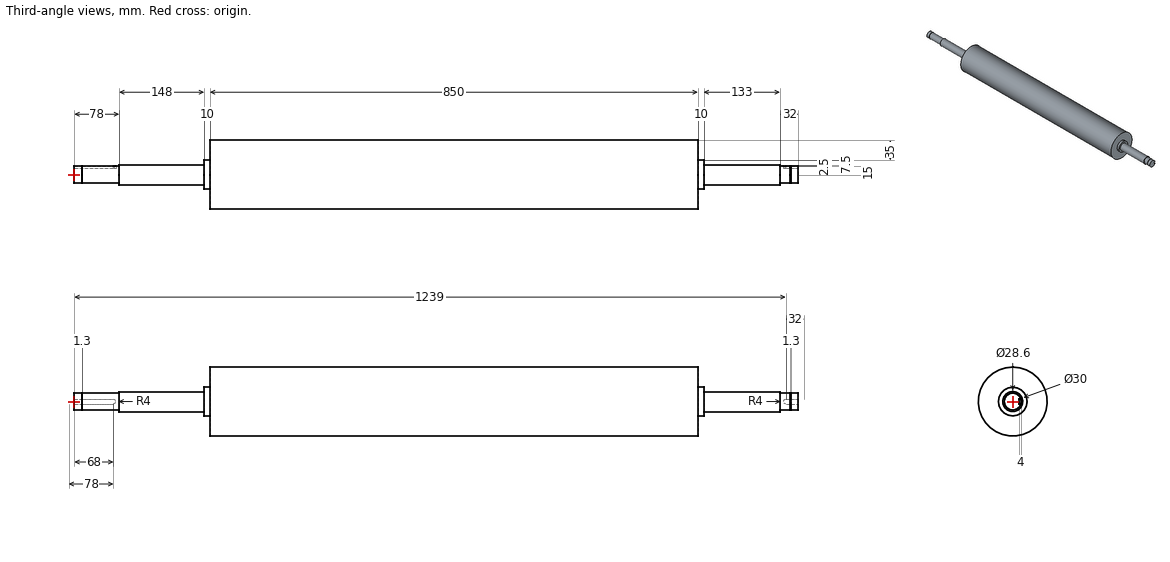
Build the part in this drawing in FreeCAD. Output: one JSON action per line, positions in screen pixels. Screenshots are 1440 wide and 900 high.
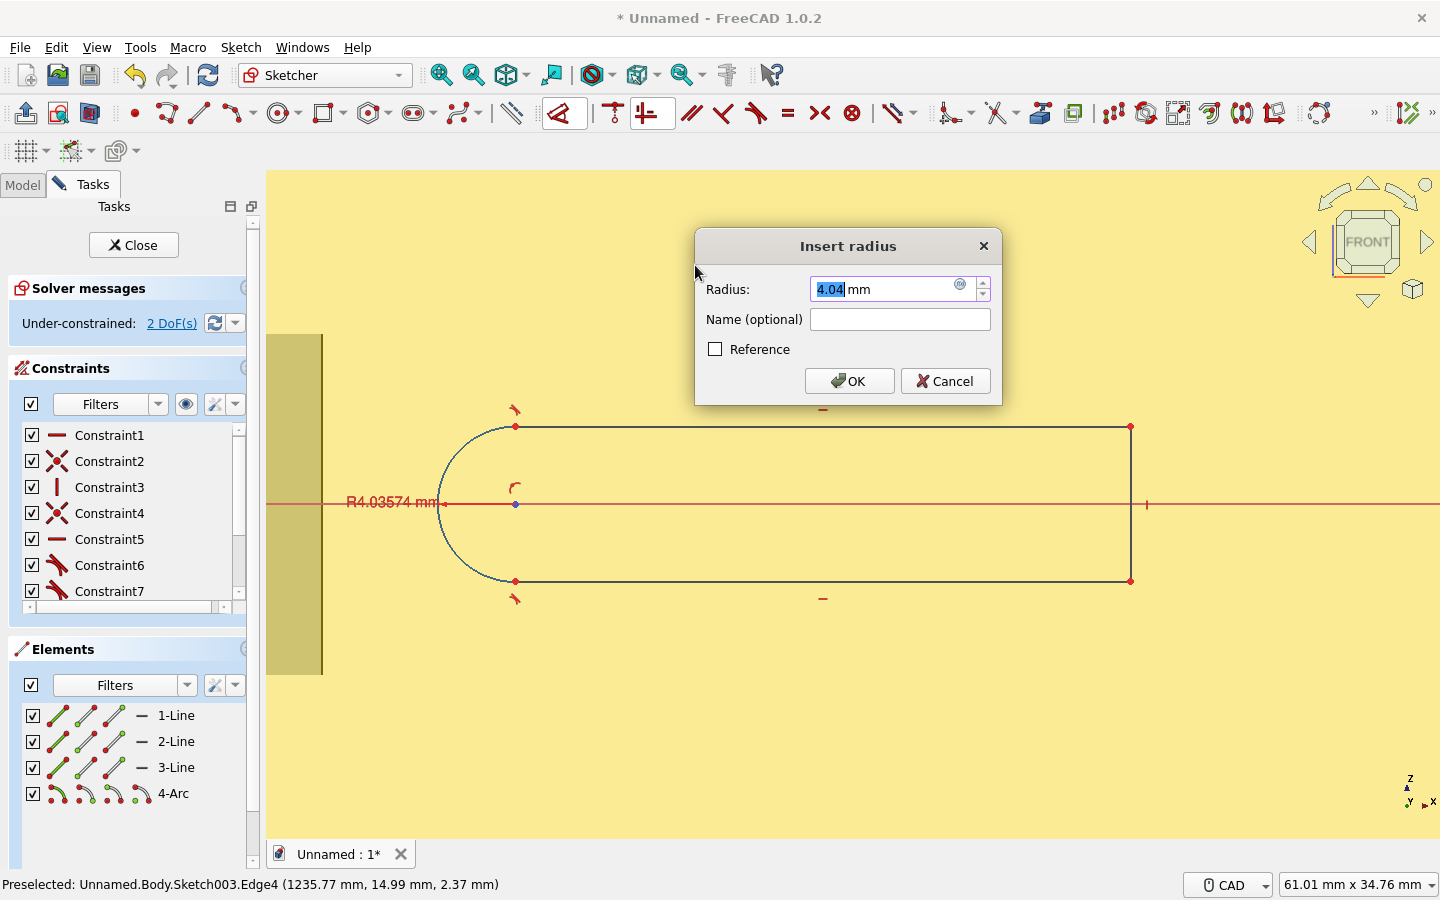
{"action": "type", "text": "4"}
{"action": "key", "text": "Return"}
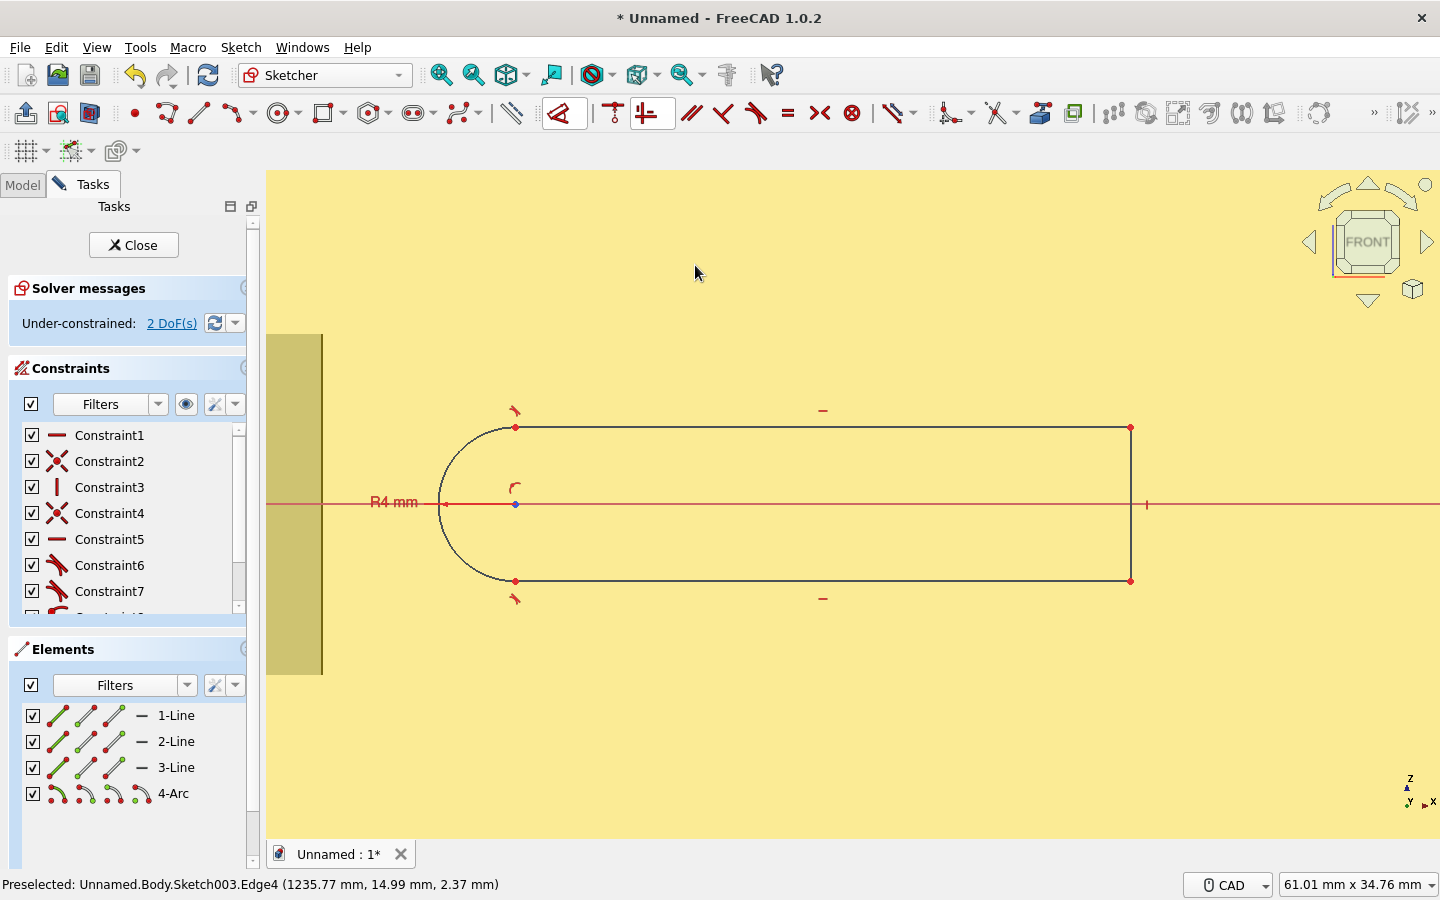
{"action": "left_click", "coordinate": [700, 427]}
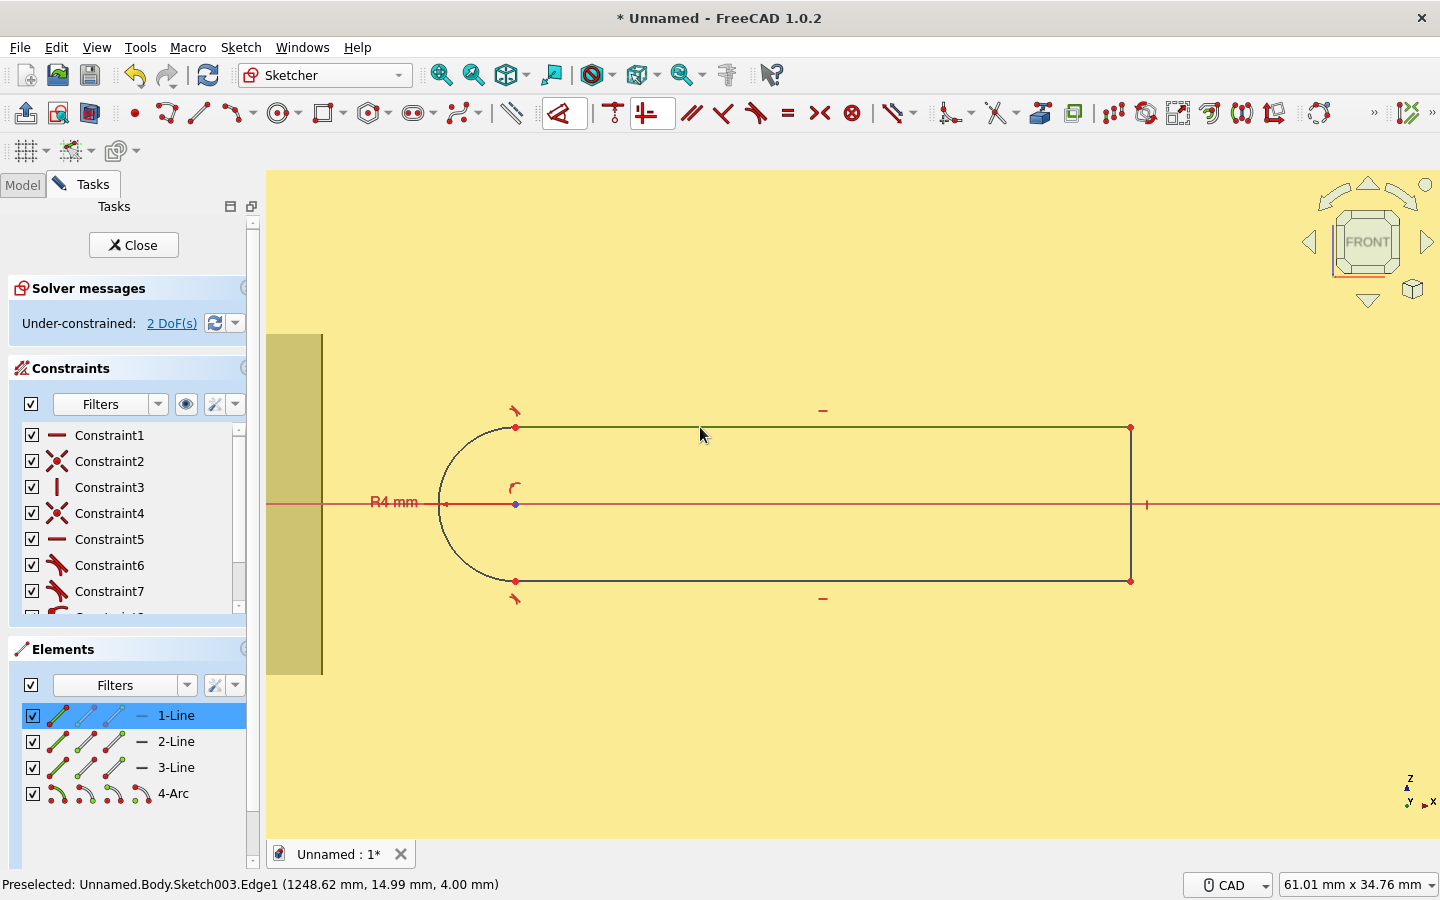
{"action": "key", "text": "l"}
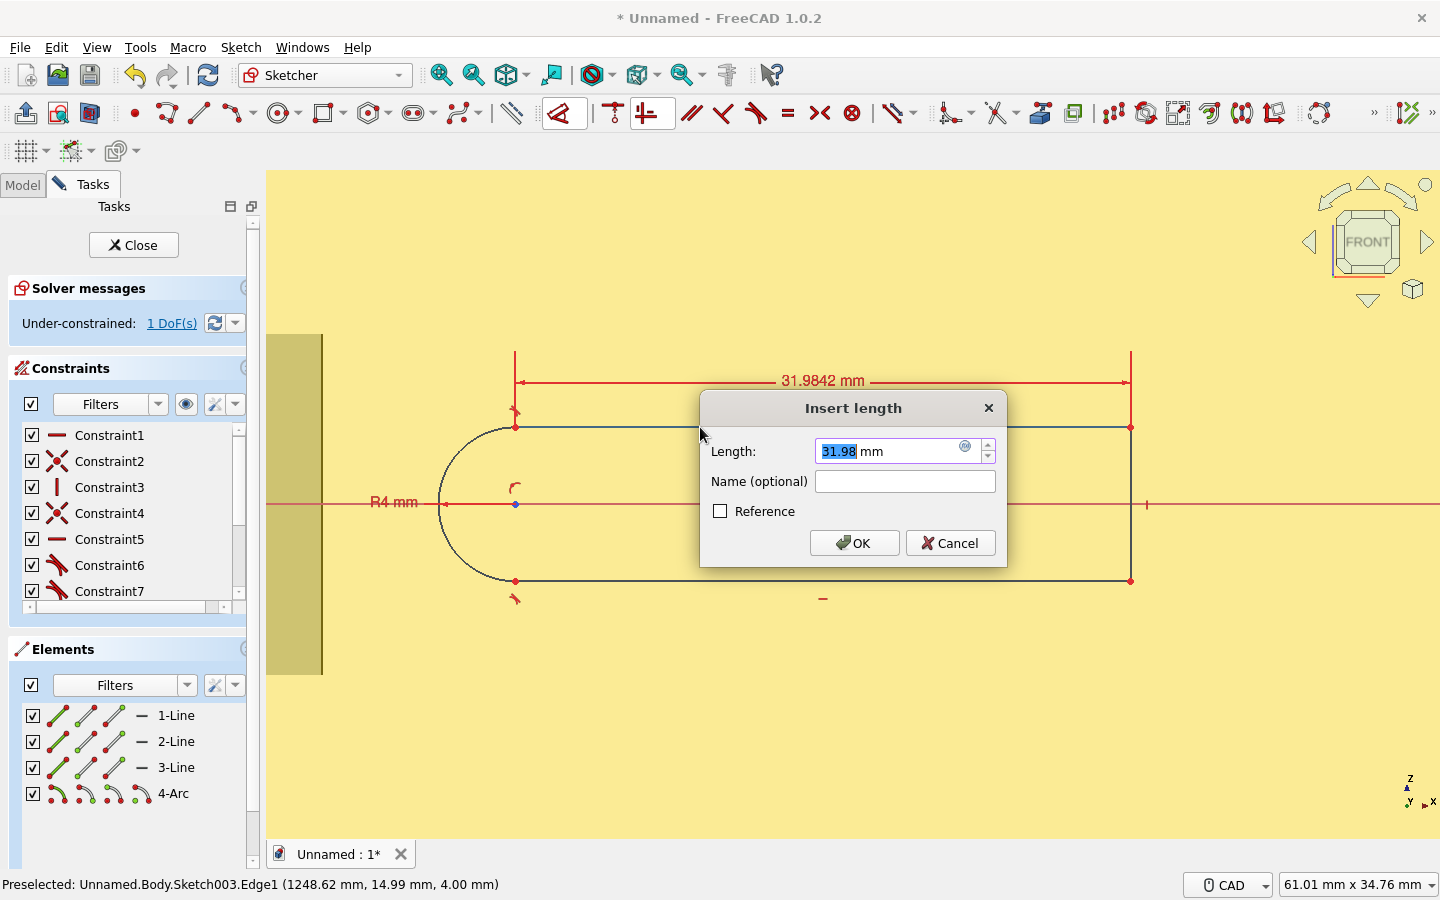
{"action": "type", "text": "32"}
{"action": "key", "text": "Return"}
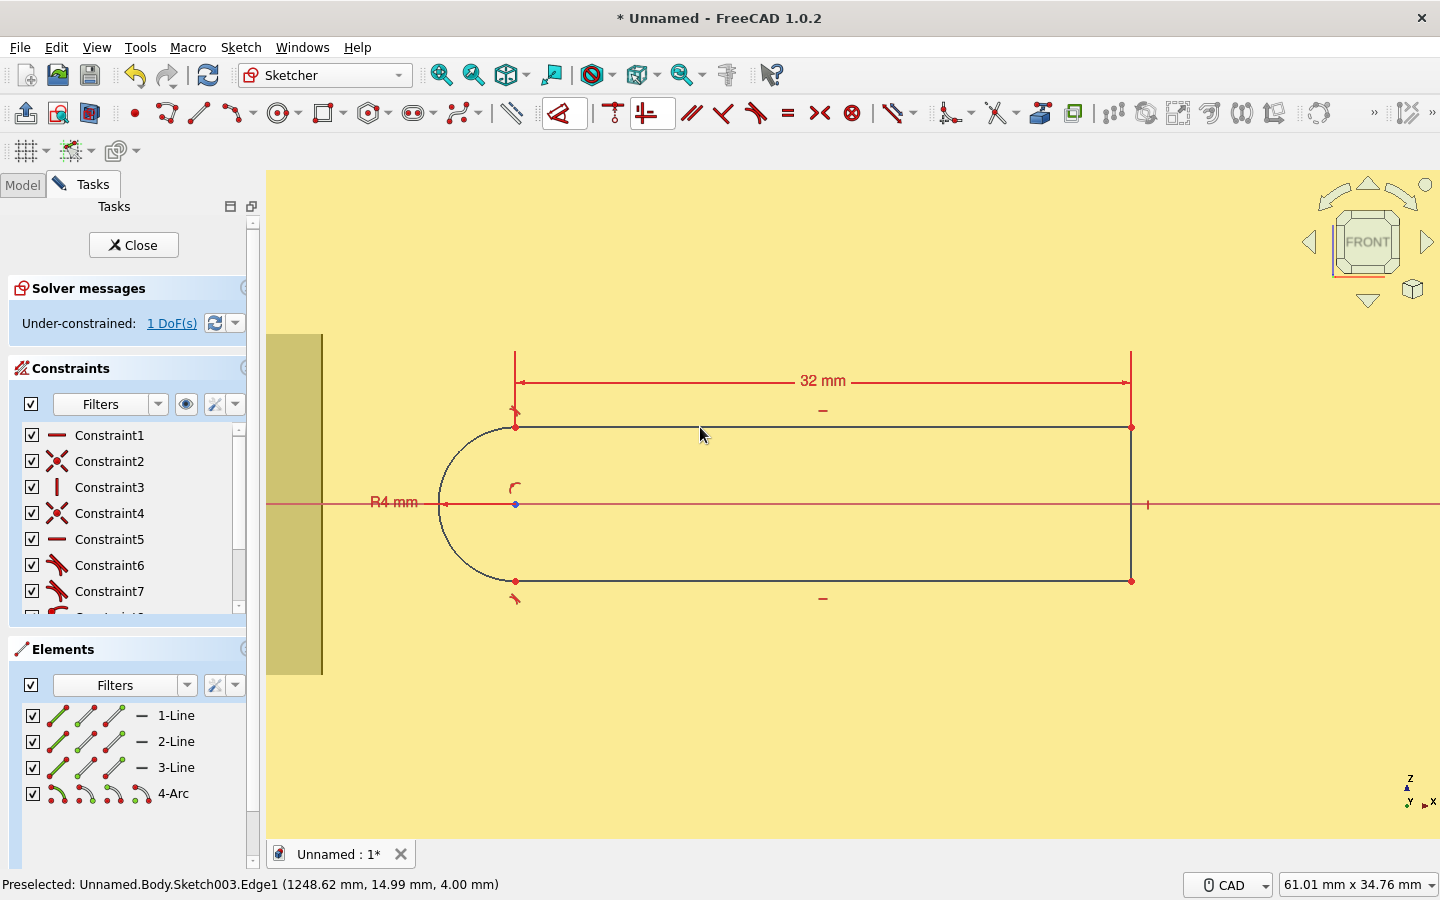
{"action": "left_click", "coordinate": [515, 427]}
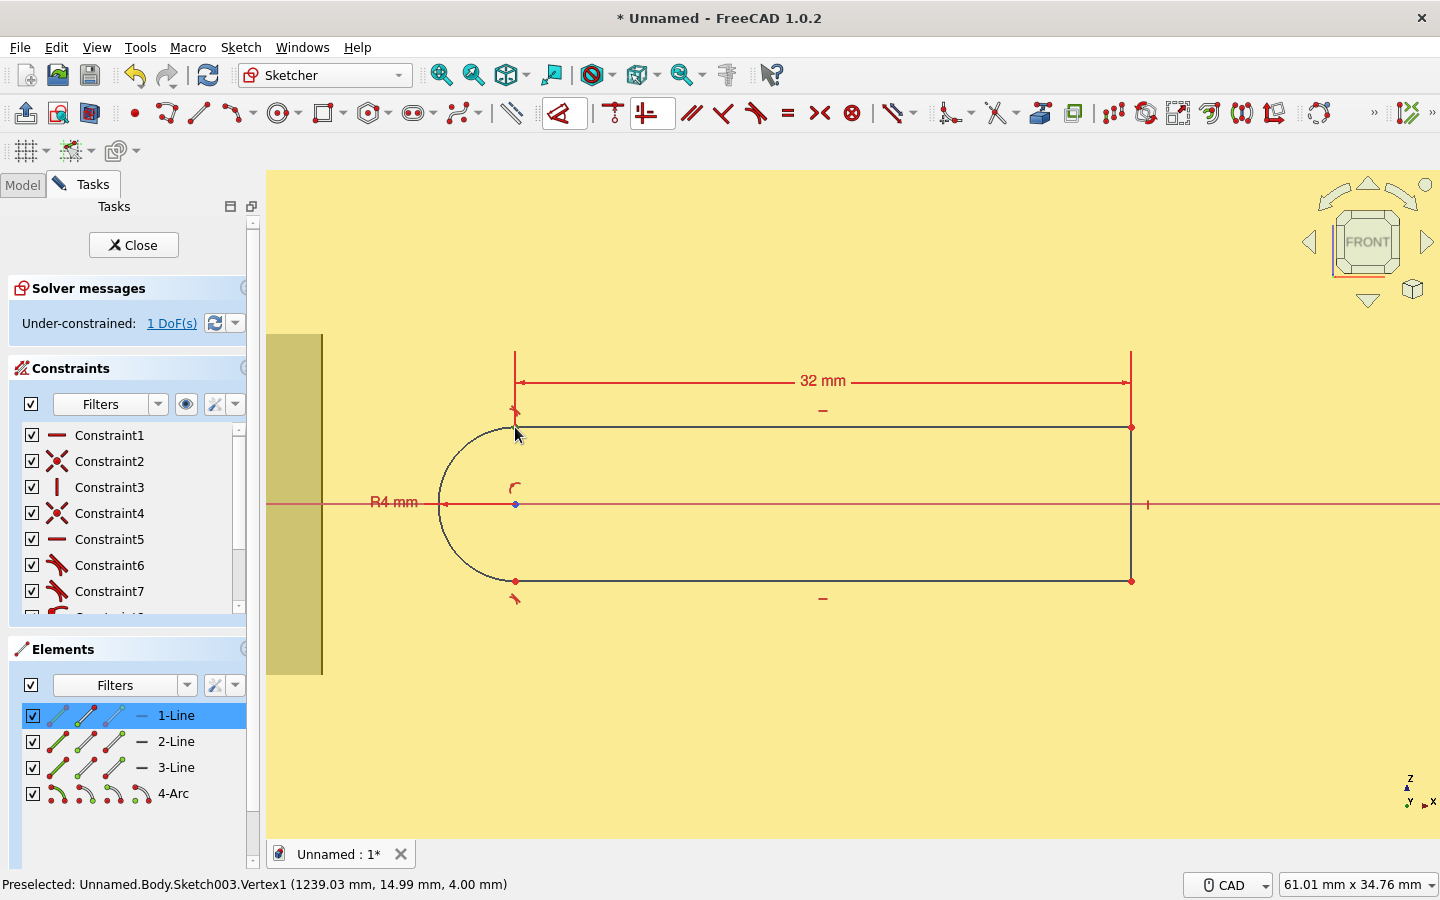
{"action": "key", "text": "l"}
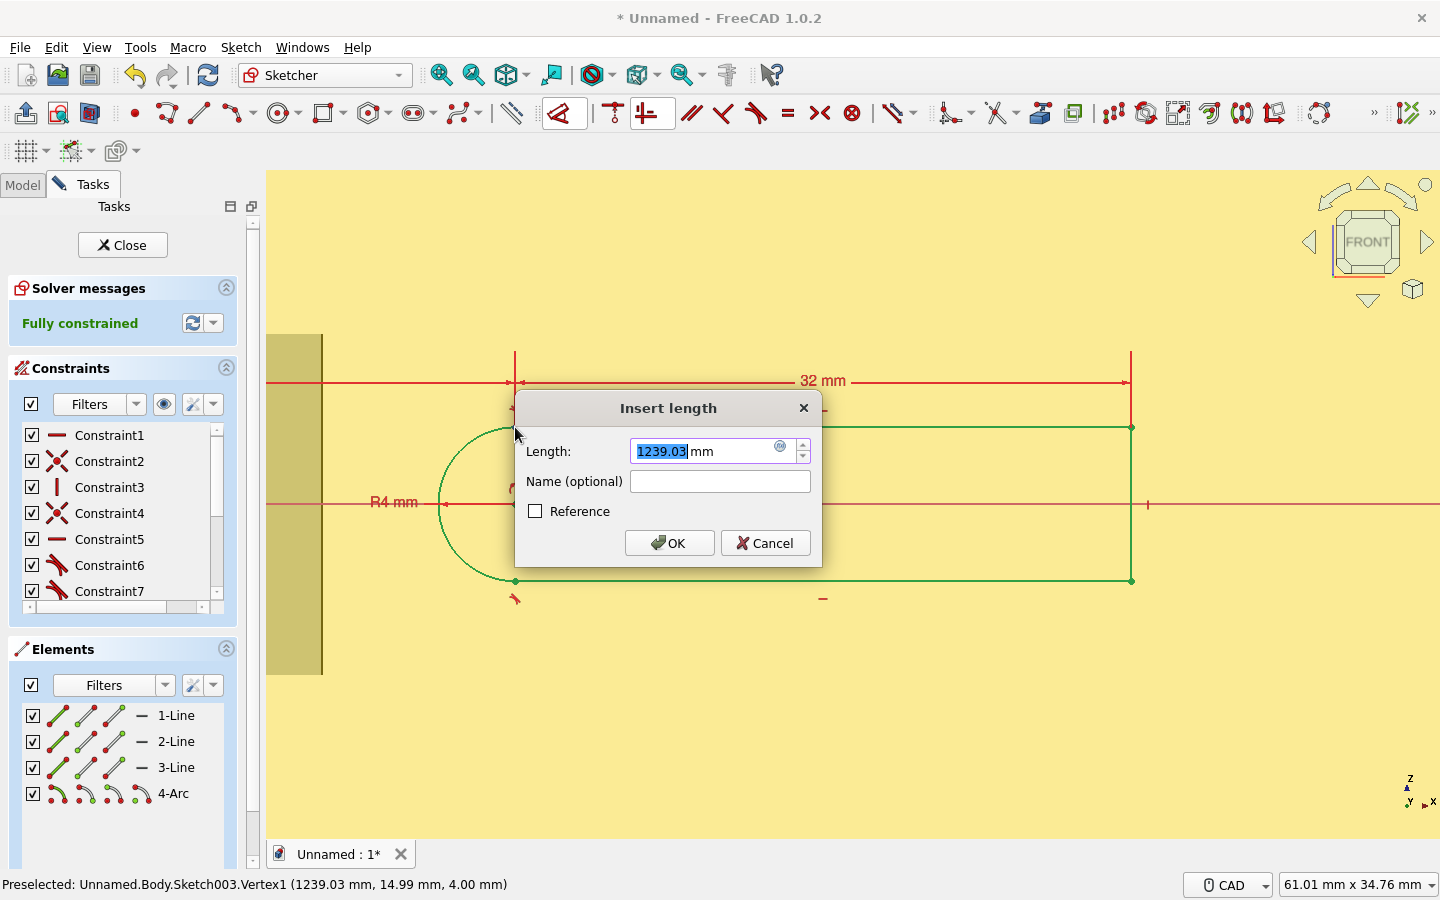
{"action": "type", "text": "1239"}
{"action": "key", "text": "Return"}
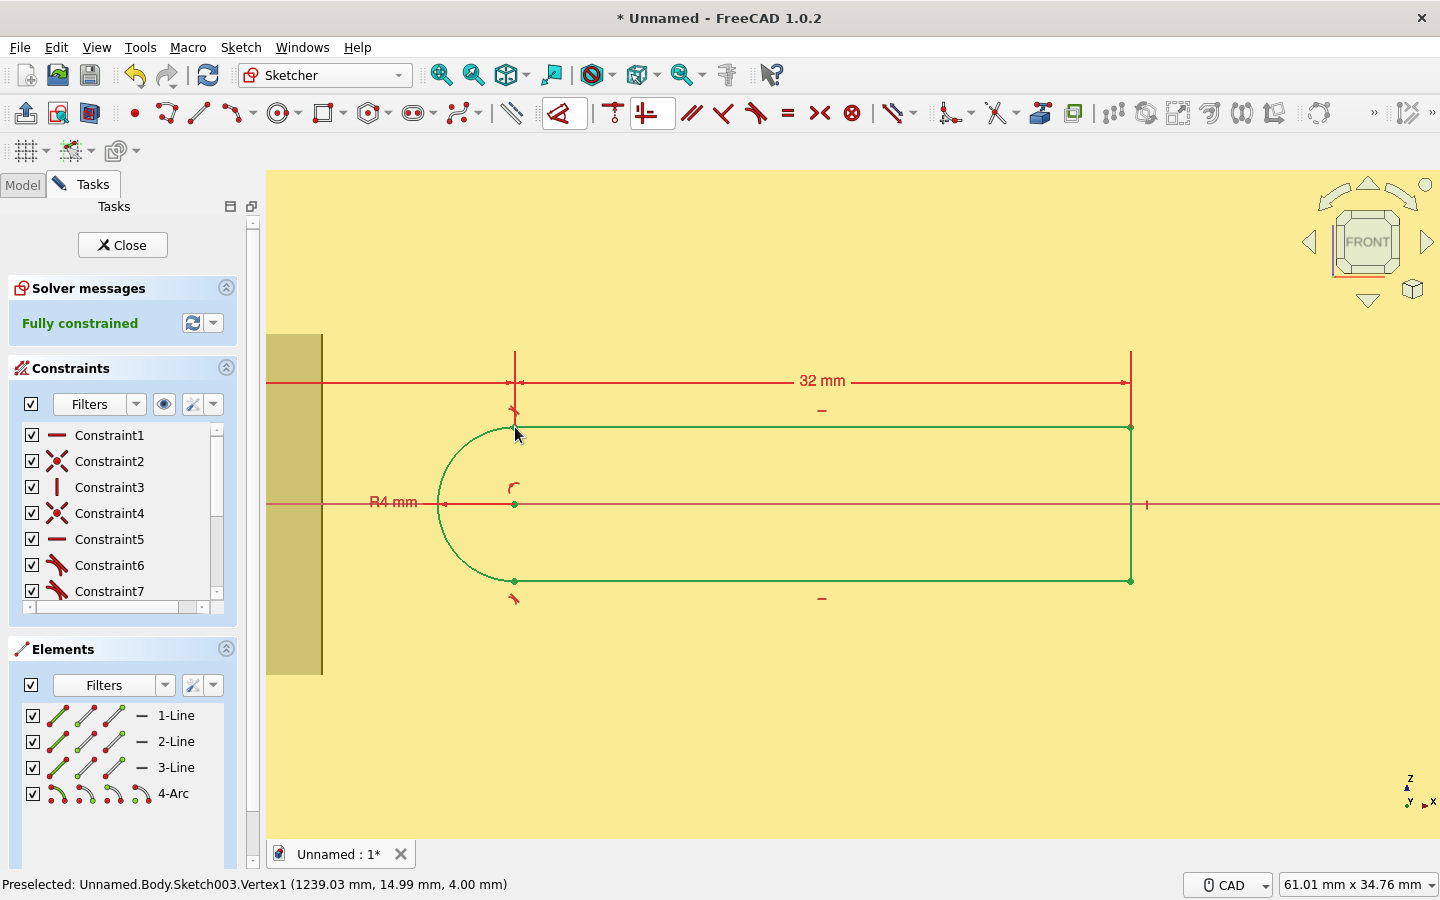
{"action": "left_click", "coordinate": [123, 245]}